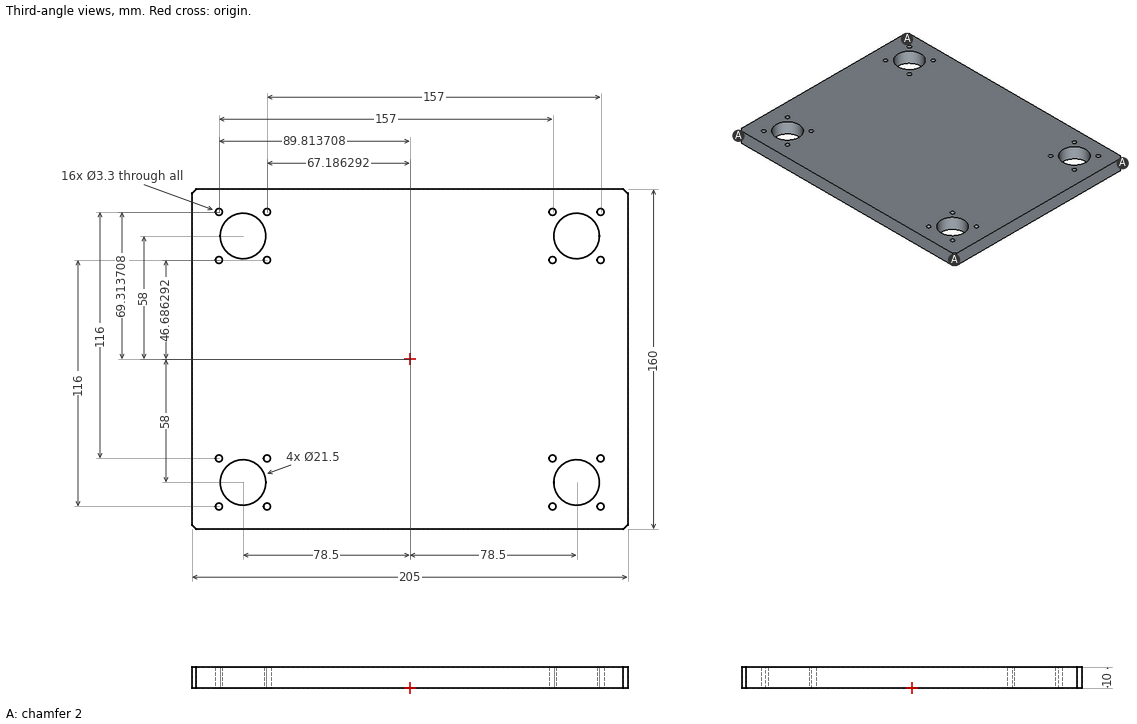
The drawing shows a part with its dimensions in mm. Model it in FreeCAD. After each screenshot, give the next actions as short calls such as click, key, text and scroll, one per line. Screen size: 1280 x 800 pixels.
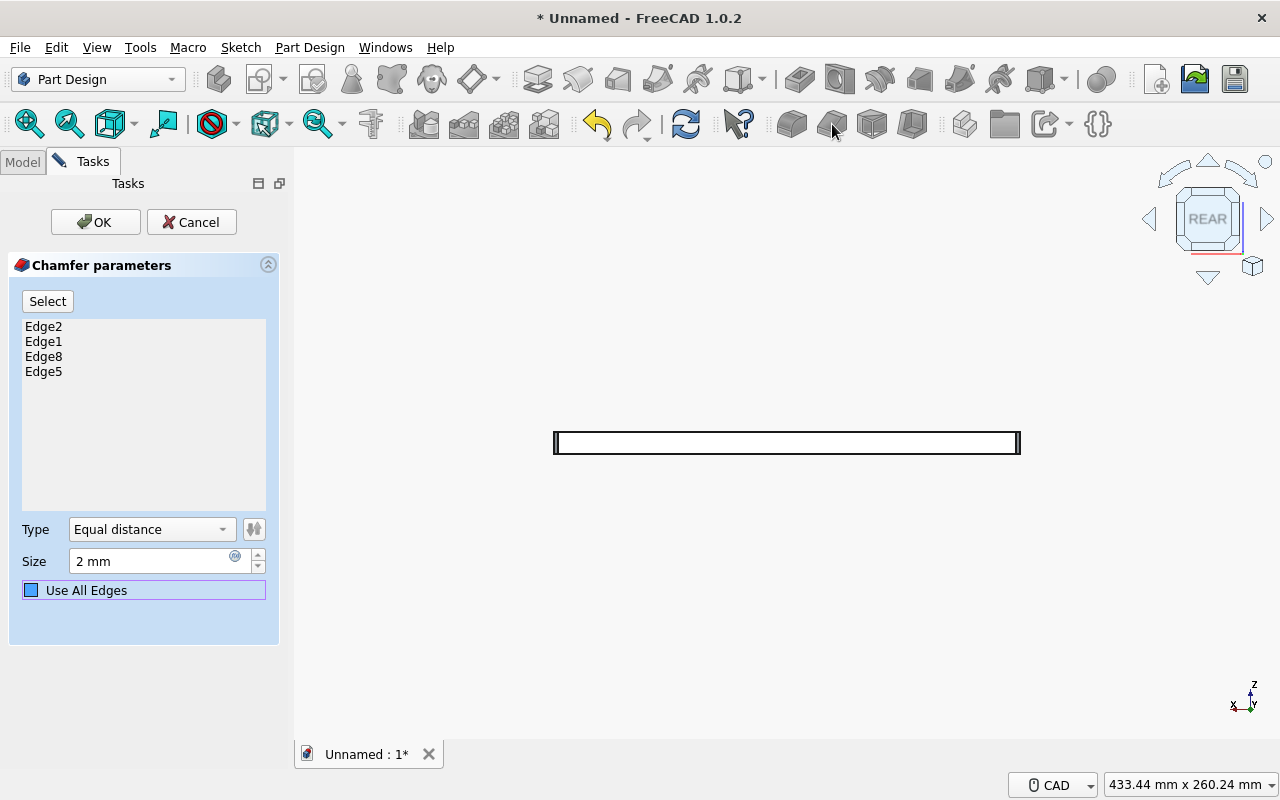
click(96, 222)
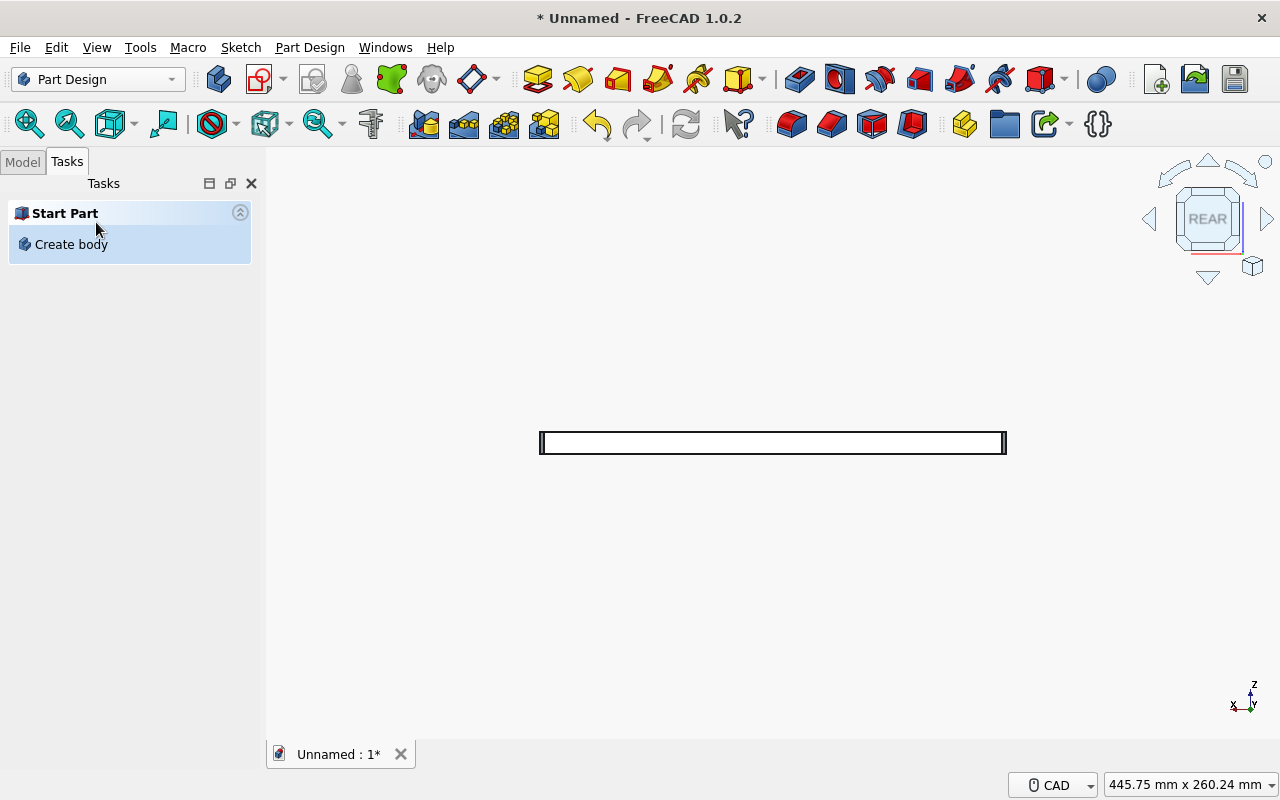
key(0)